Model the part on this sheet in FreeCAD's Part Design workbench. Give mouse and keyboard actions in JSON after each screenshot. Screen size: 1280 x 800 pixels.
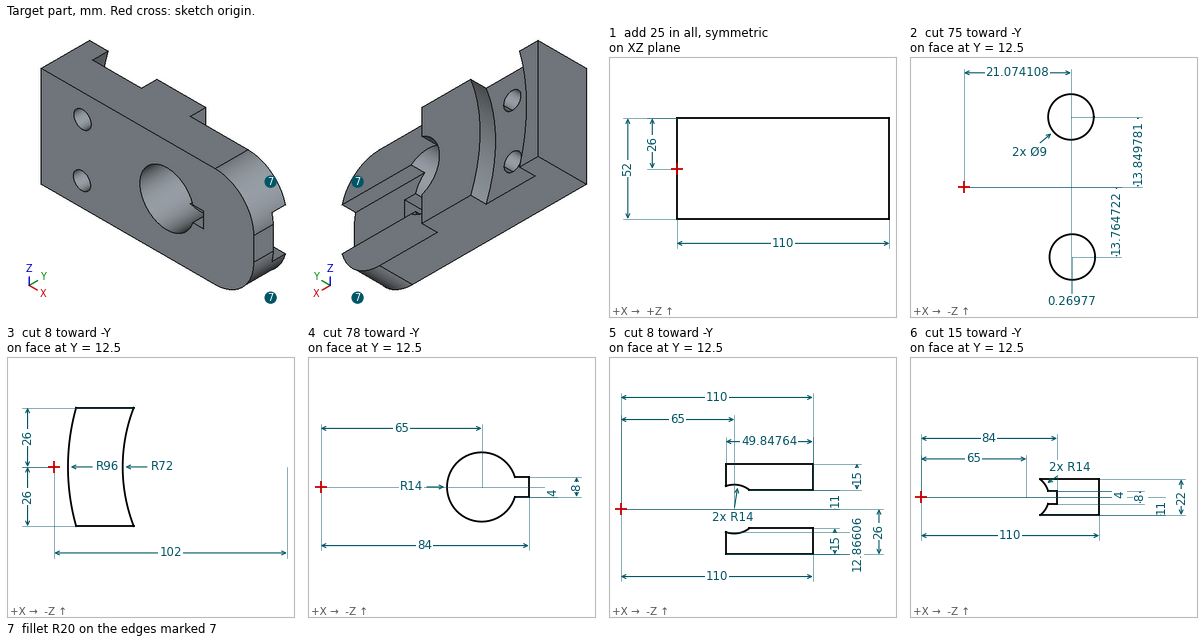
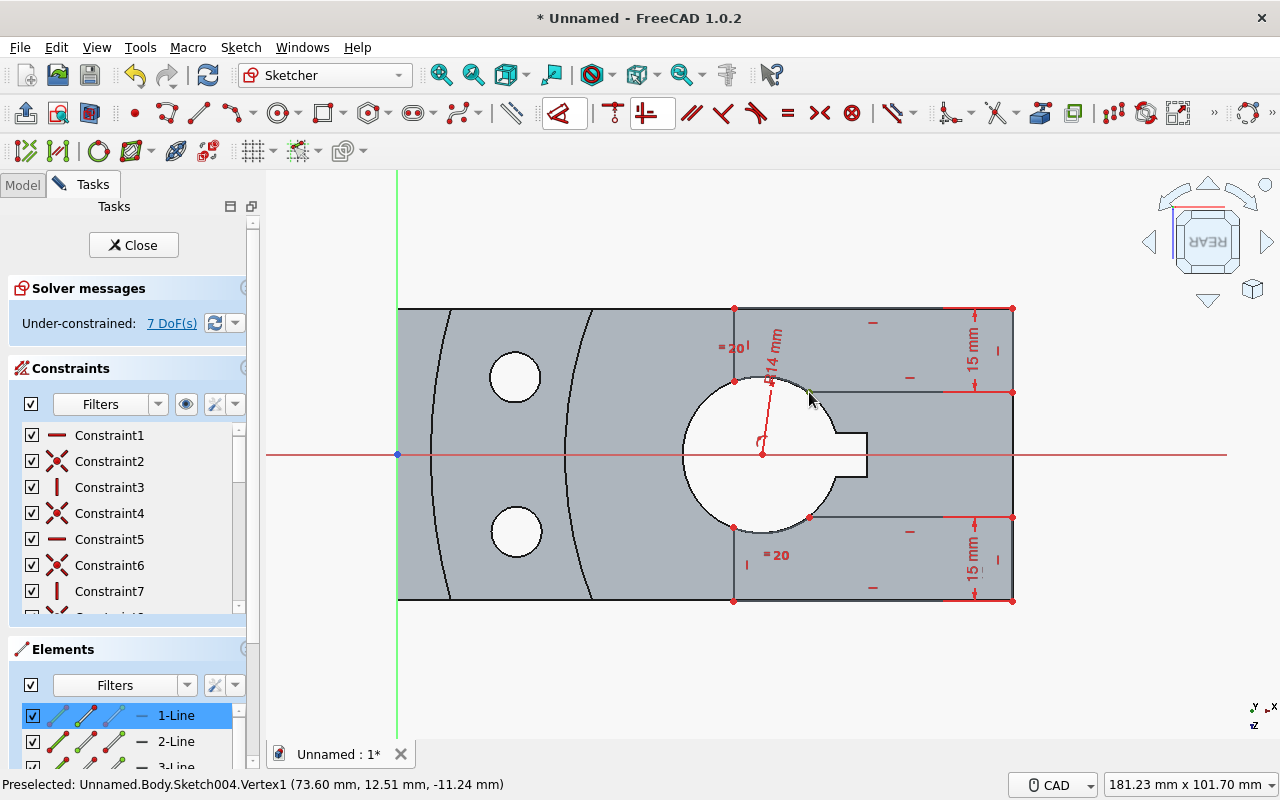
{"action": "left_click", "coordinate": [582, 114]}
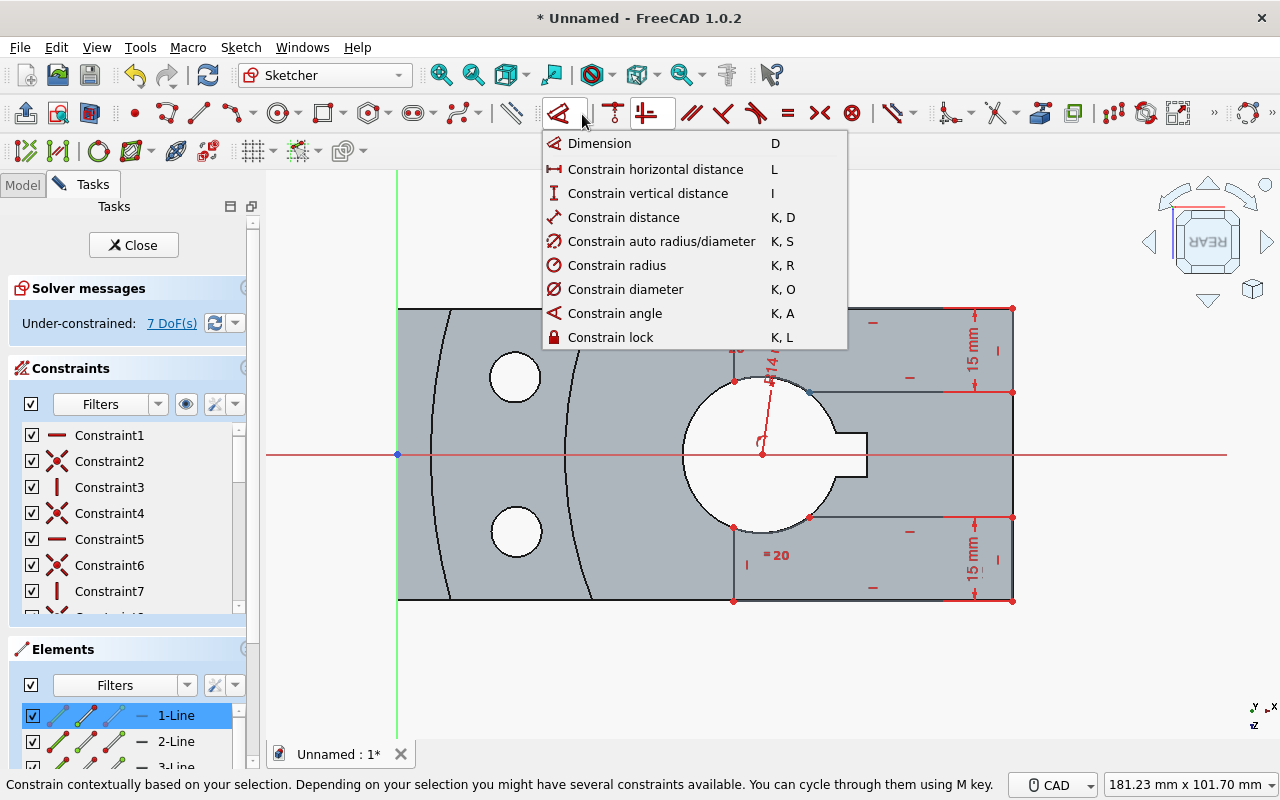
{"action": "left_click", "coordinate": [695, 193]}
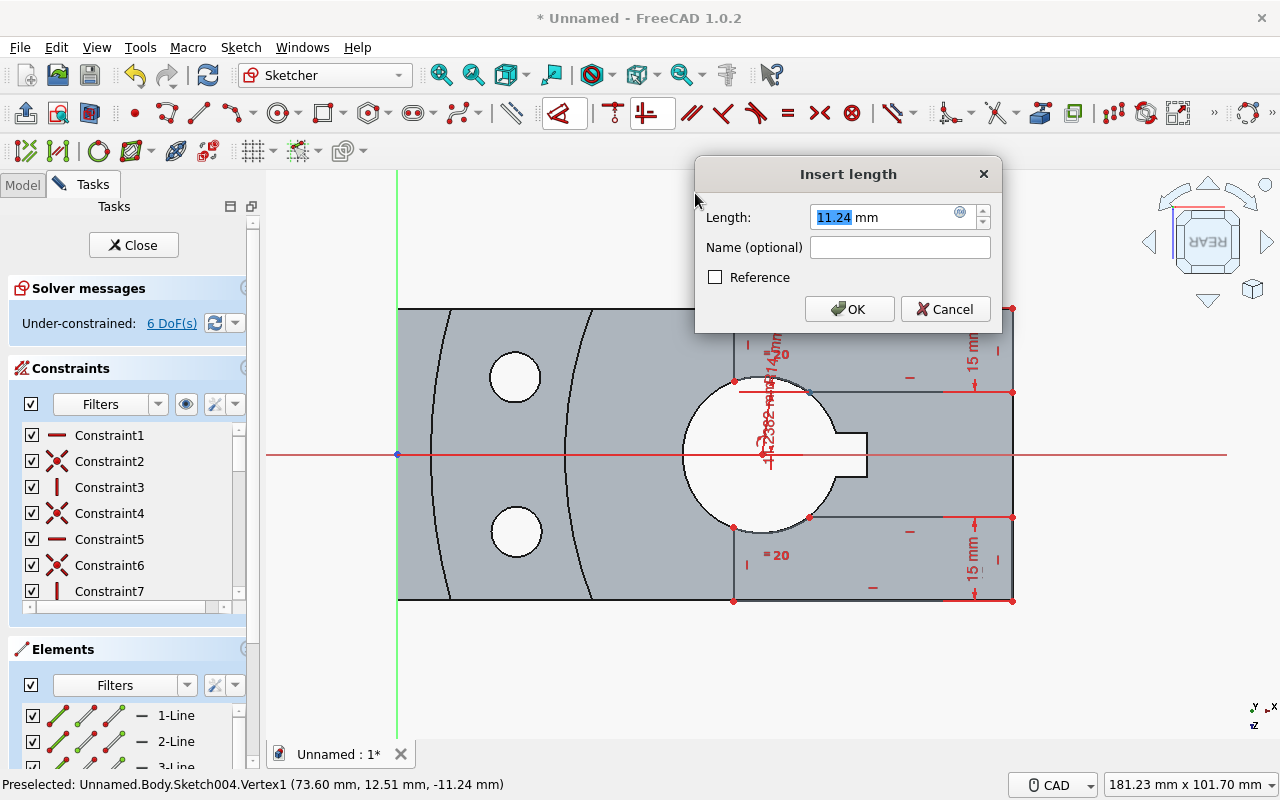
{"action": "type", "text": "11"}
{"action": "key", "text": "Return"}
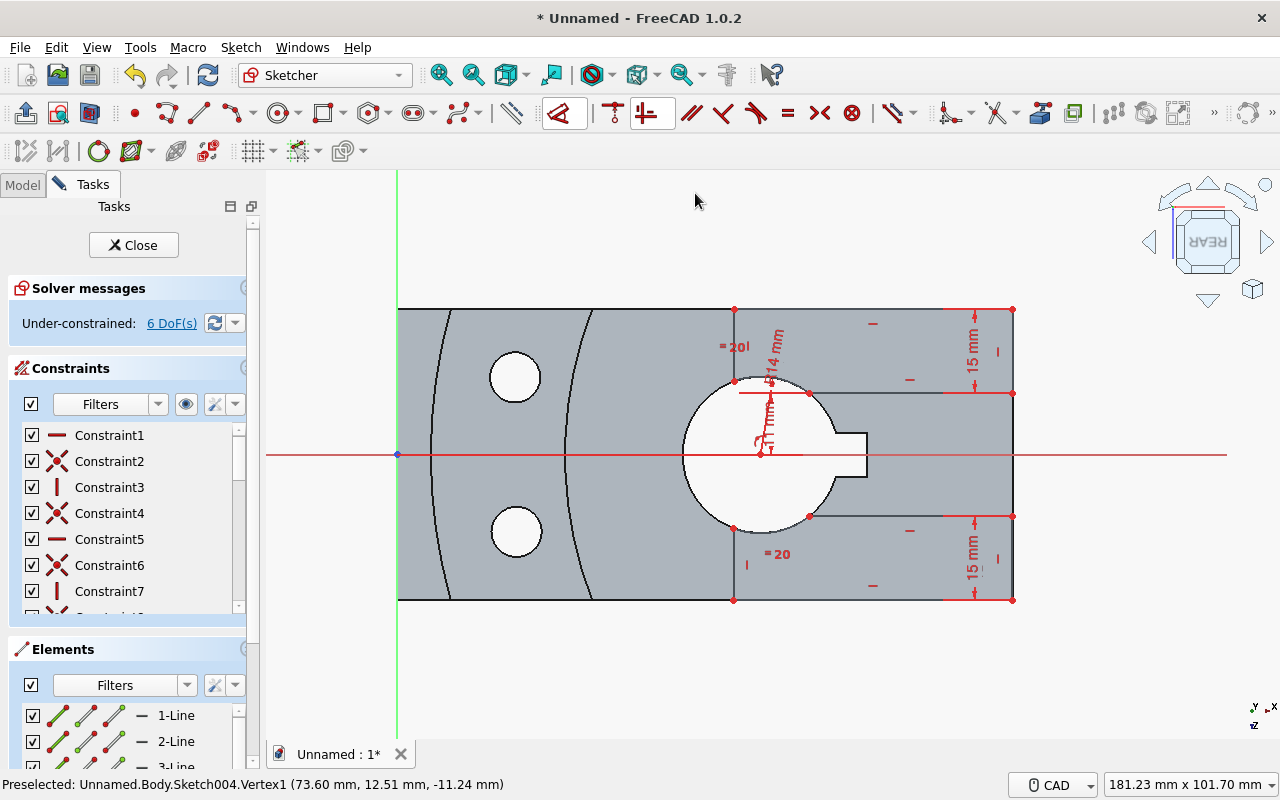
{"action": "left_click", "coordinate": [734, 600]}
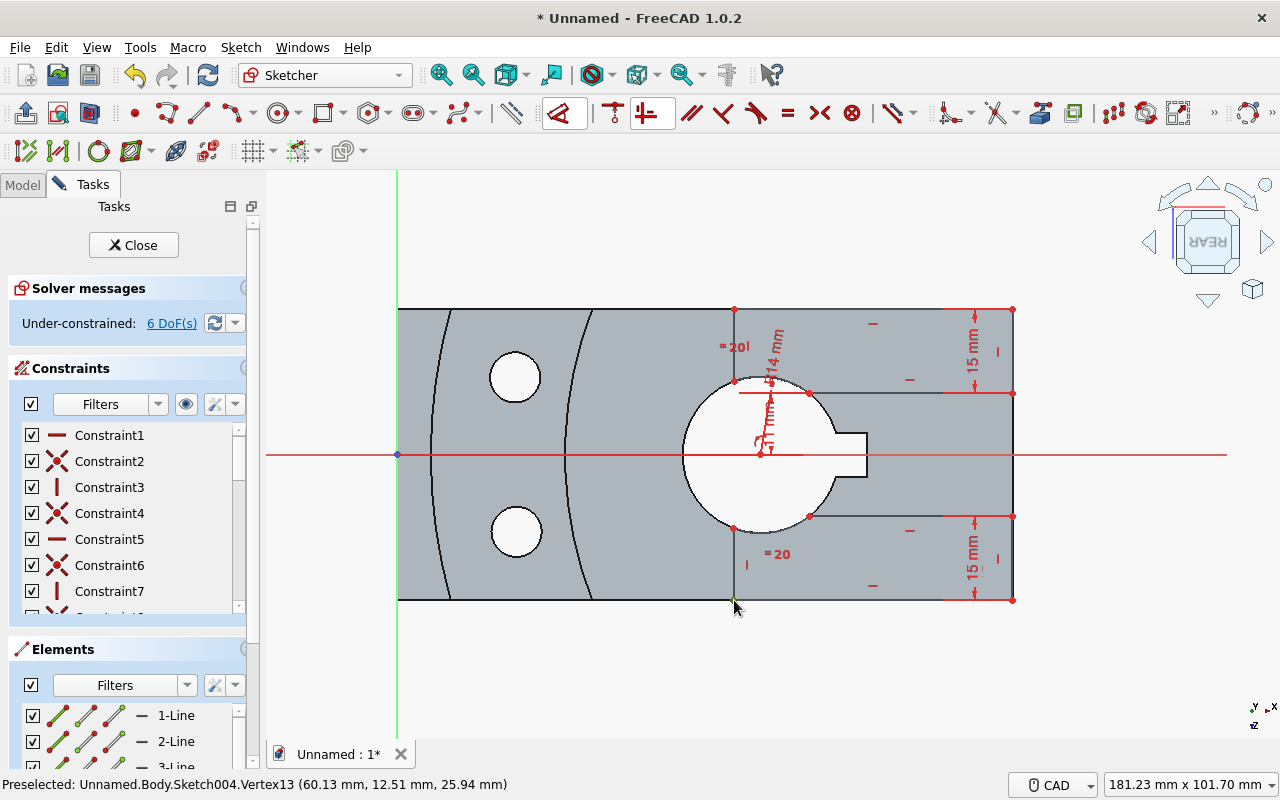
{"action": "left_click", "coordinate": [582, 114]}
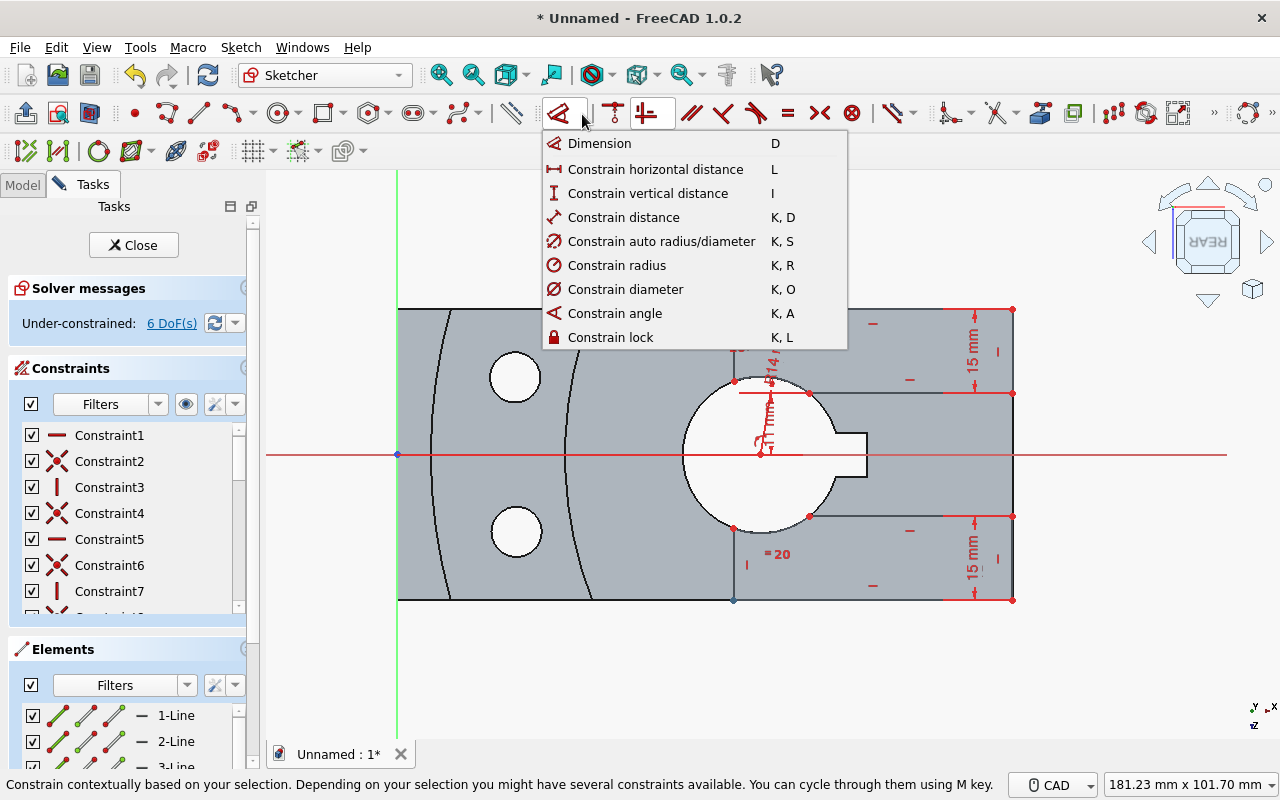
{"action": "left_click", "coordinate": [695, 193]}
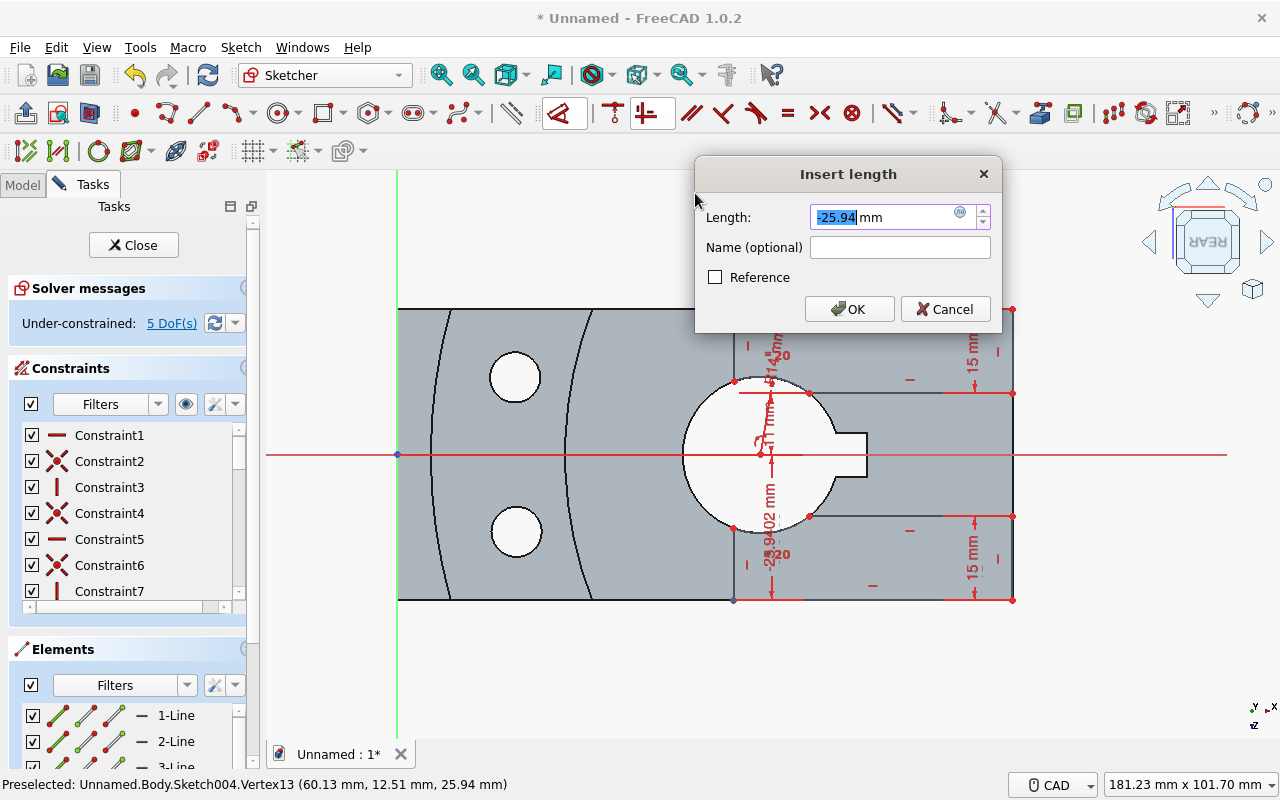
{"action": "type", "text": "-26"}
{"action": "key", "text": "Return"}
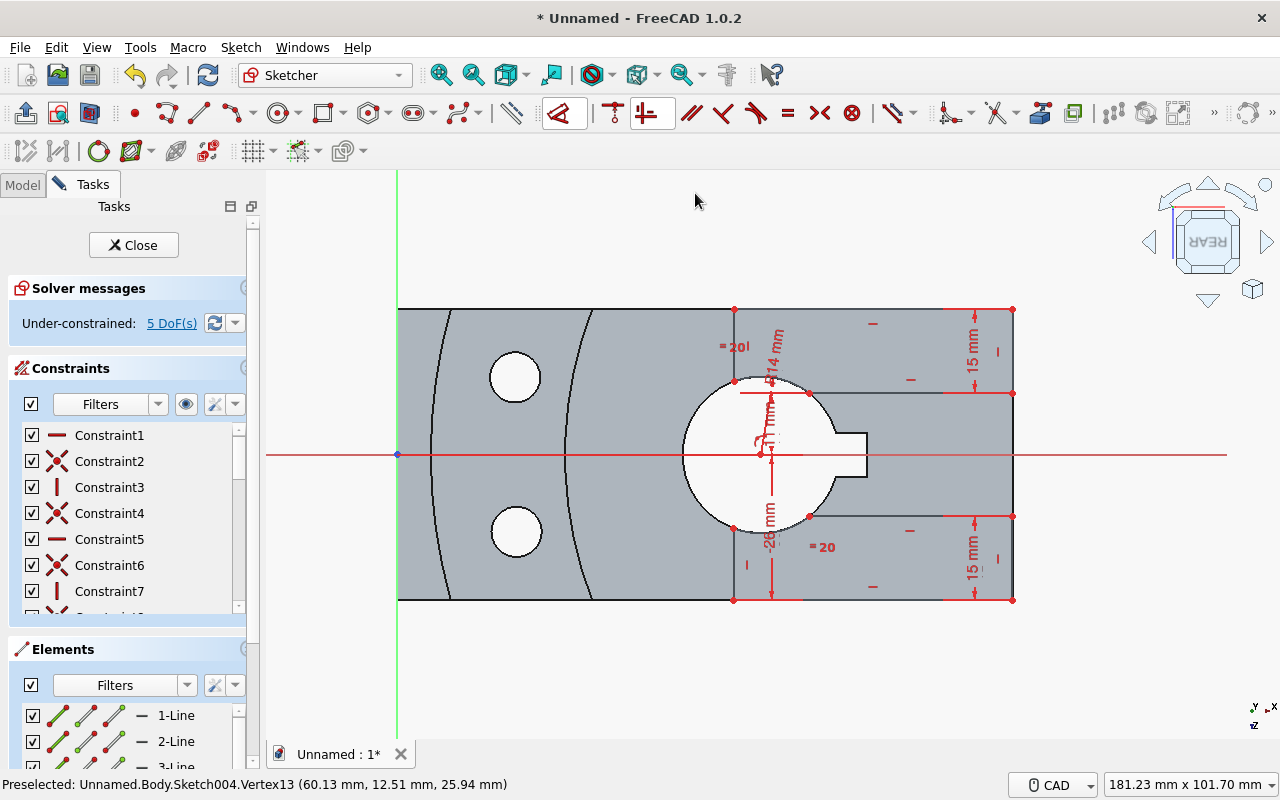
{"action": "left_click", "coordinate": [761, 455]}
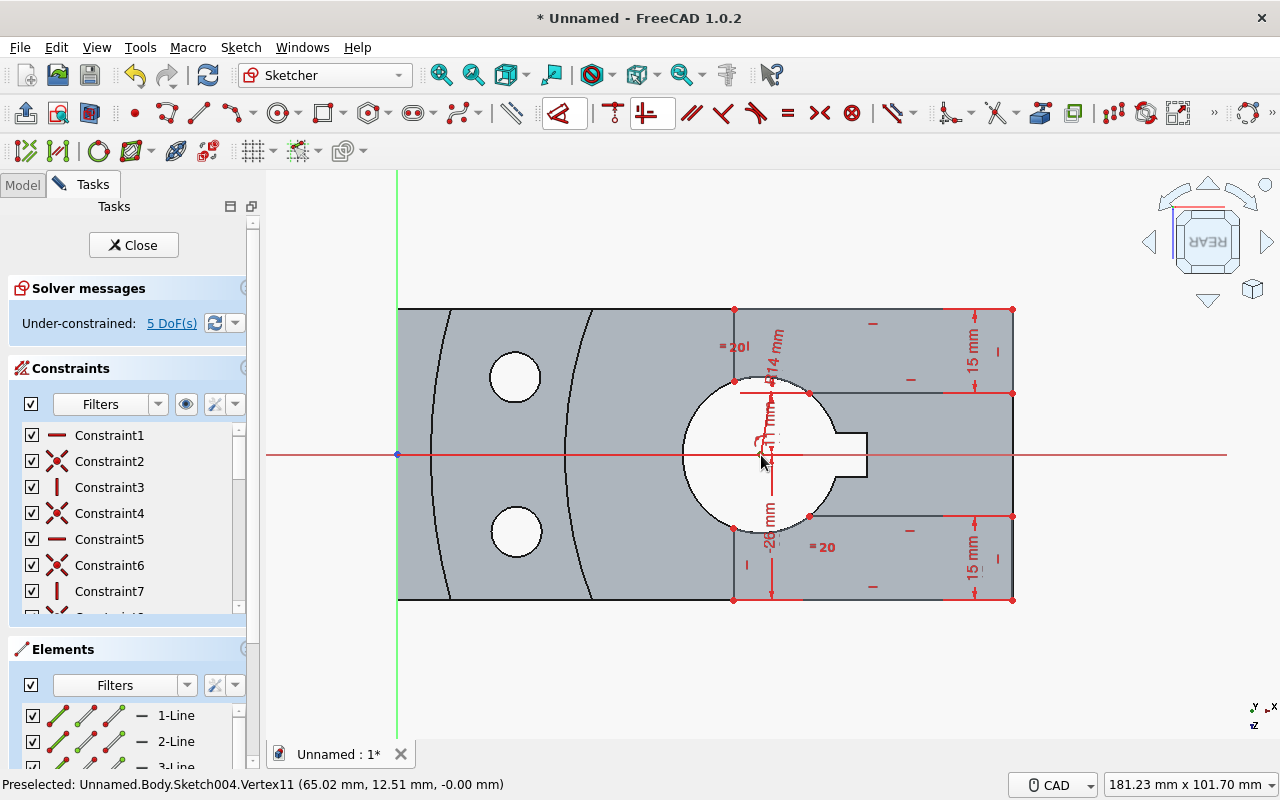
{"action": "key", "text": "l"}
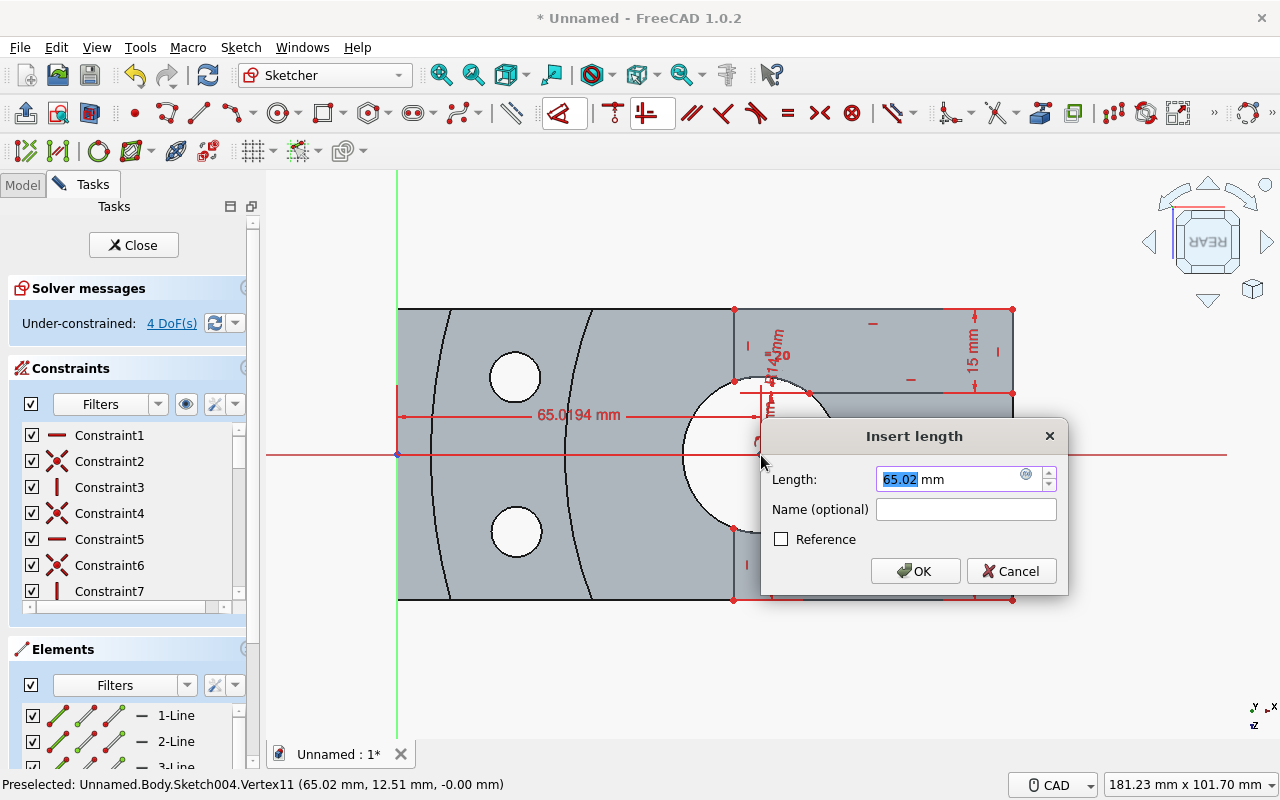
{"action": "type", "text": "65"}
{"action": "key", "text": "Return"}